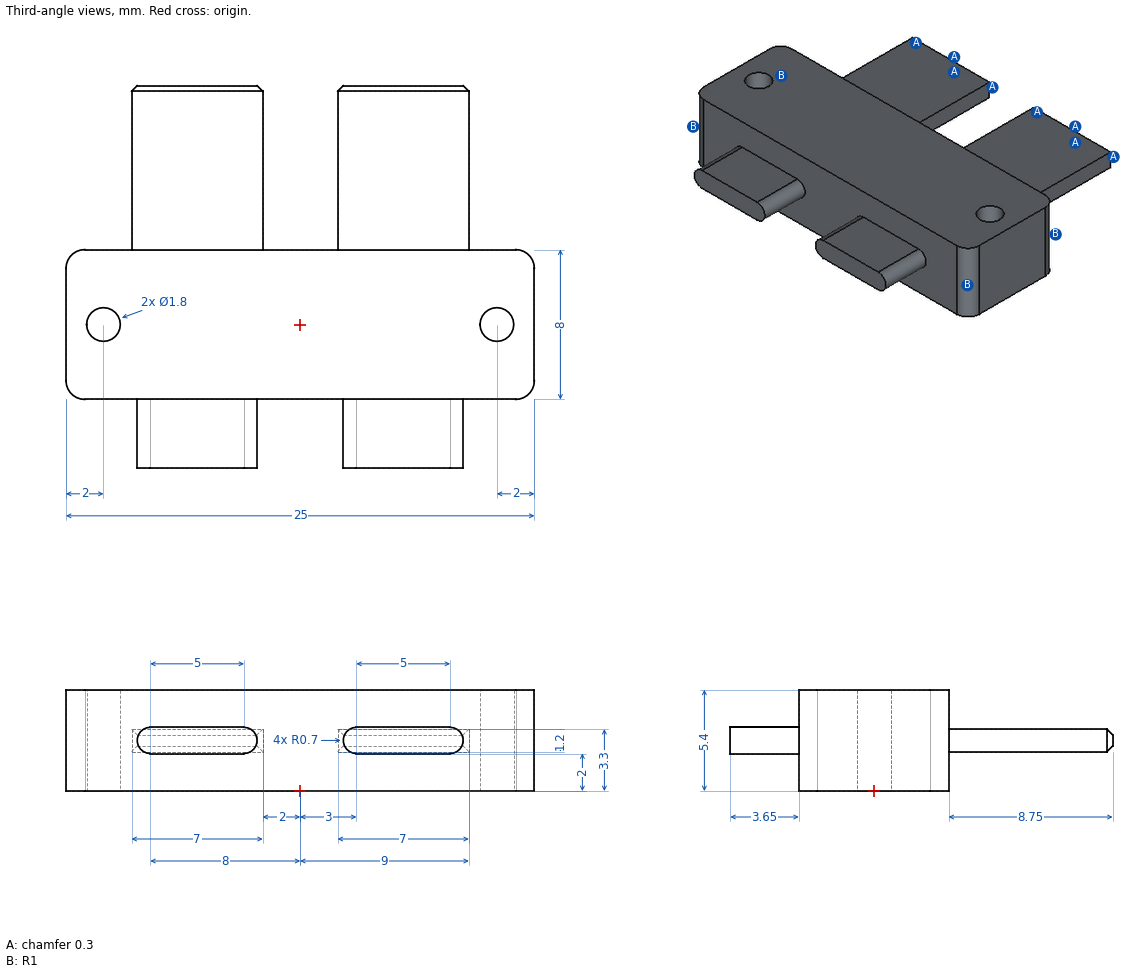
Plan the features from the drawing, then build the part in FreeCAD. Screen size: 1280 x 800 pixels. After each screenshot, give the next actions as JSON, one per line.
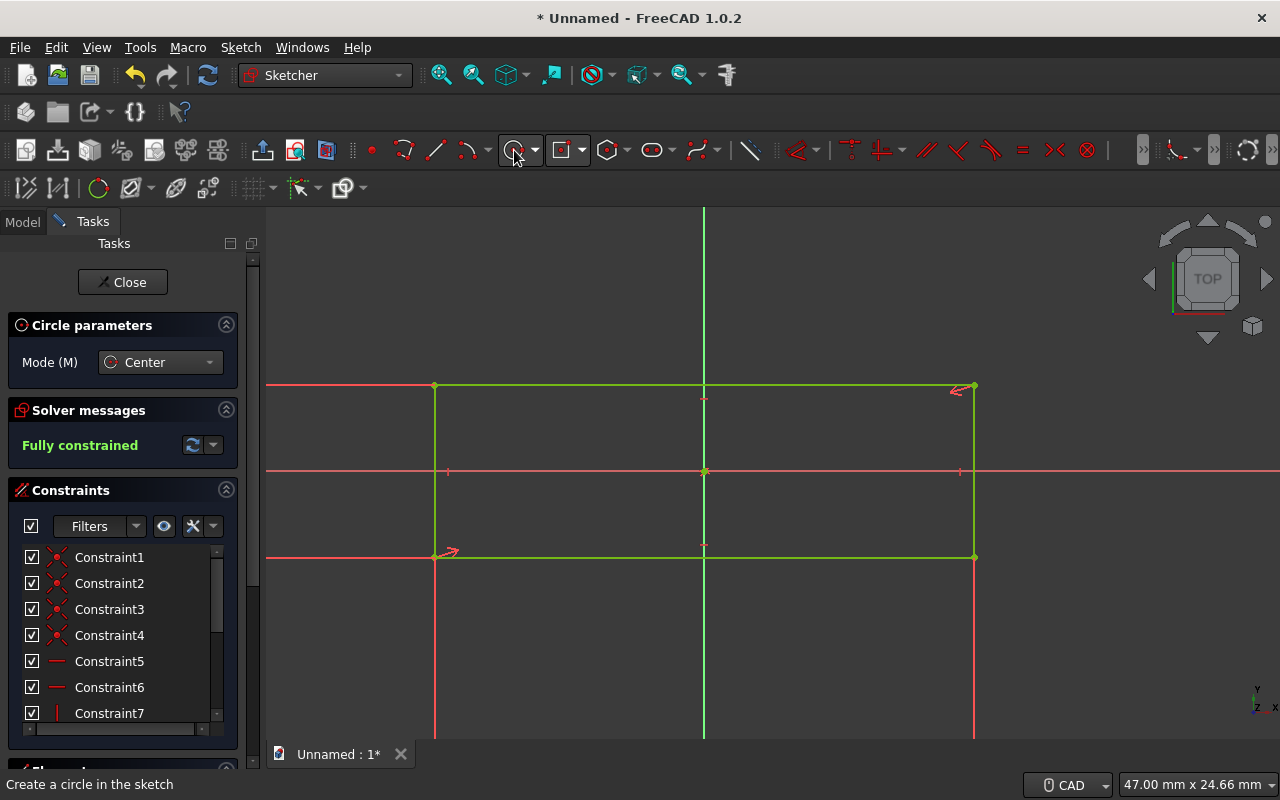
{"action": "left_click", "coordinate": [478, 471]}
{"action": "mouse_move", "coordinate": [485, 453]}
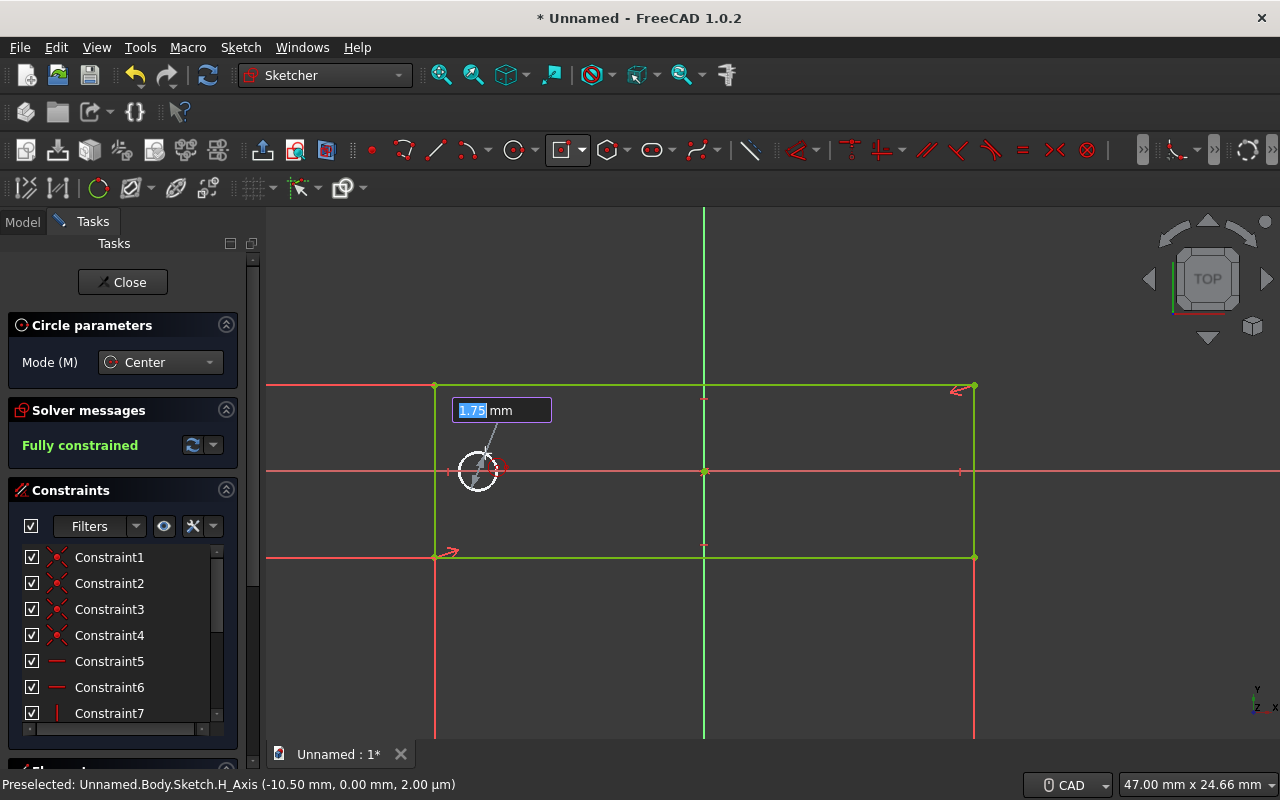
{"action": "type", "text": "1.8"}
{"action": "key", "text": "Return"}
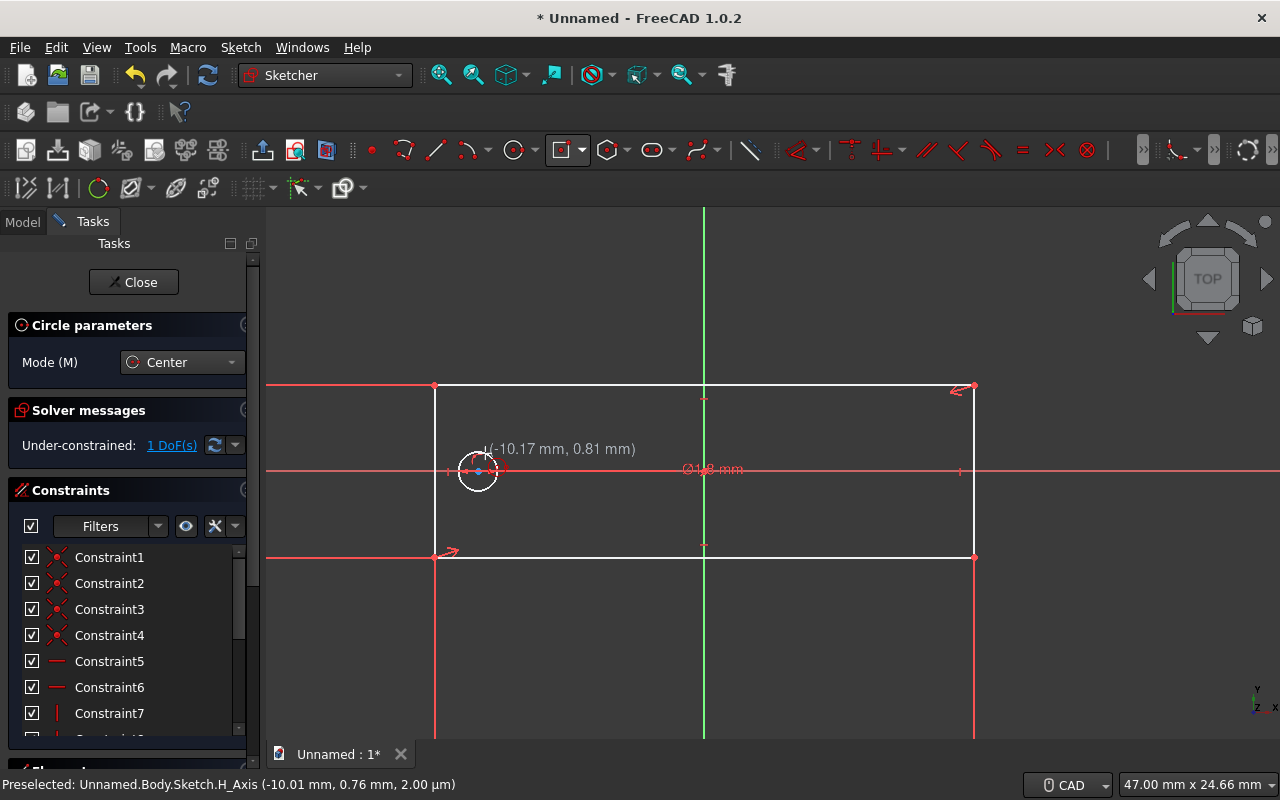
{"action": "left_click", "coordinate": [931, 471]}
{"action": "mouse_move", "coordinate": [938, 453]}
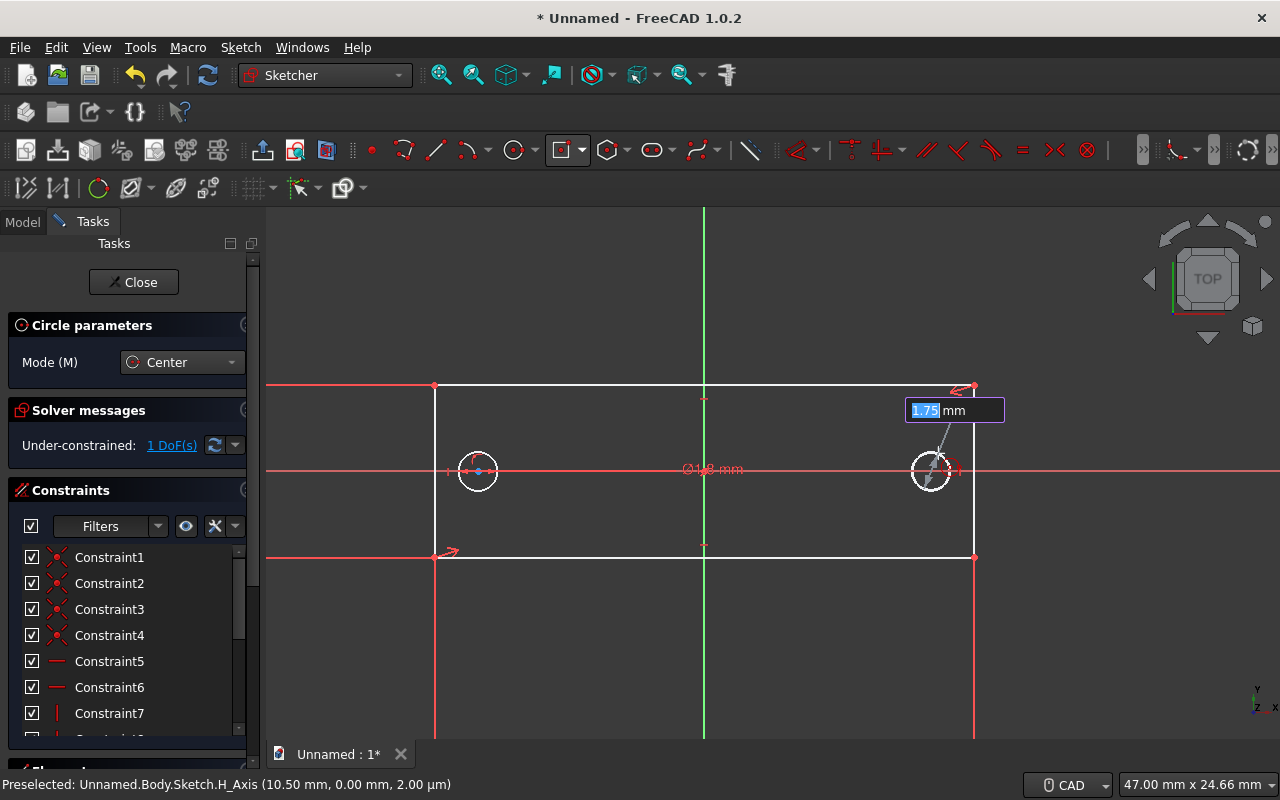
{"action": "type", "text": "1.8"}
{"action": "key", "text": "Return"}
{"action": "key", "text": "Escape"}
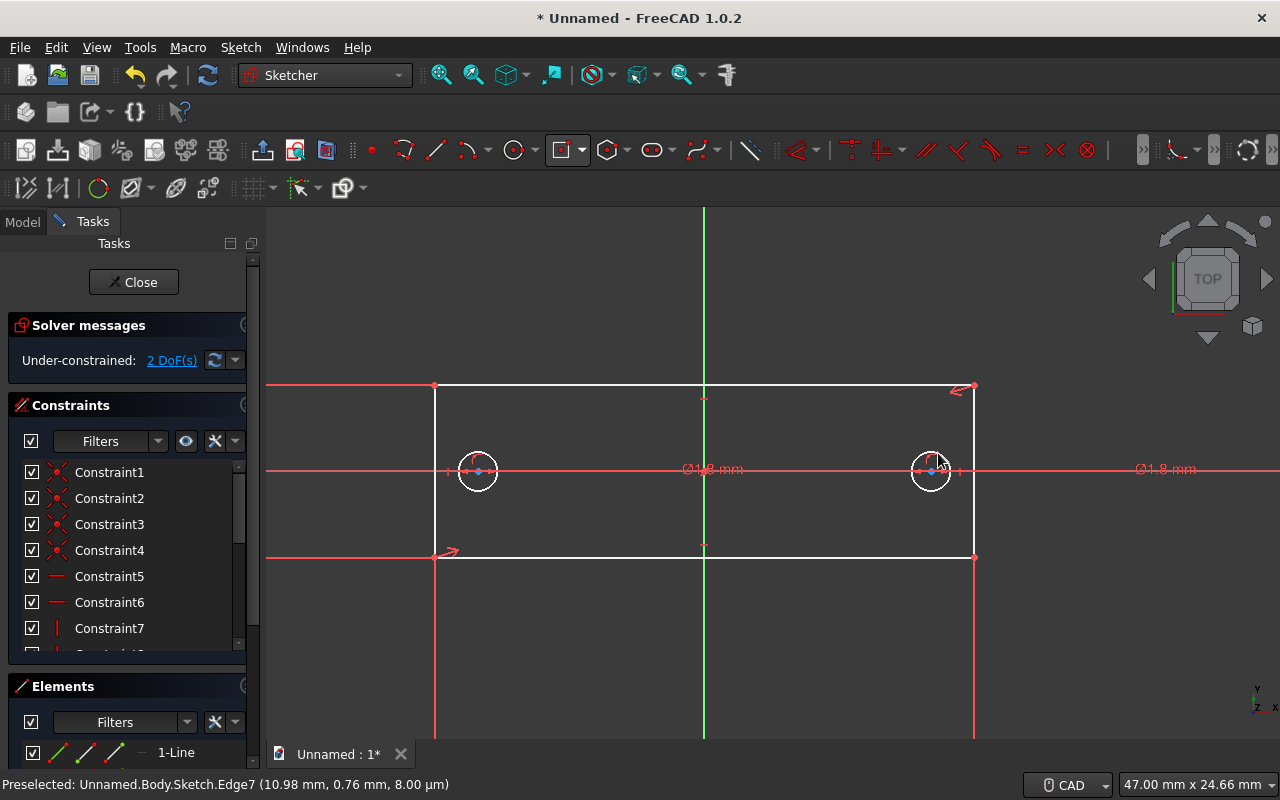
{"action": "left_click", "coordinate": [435, 558]}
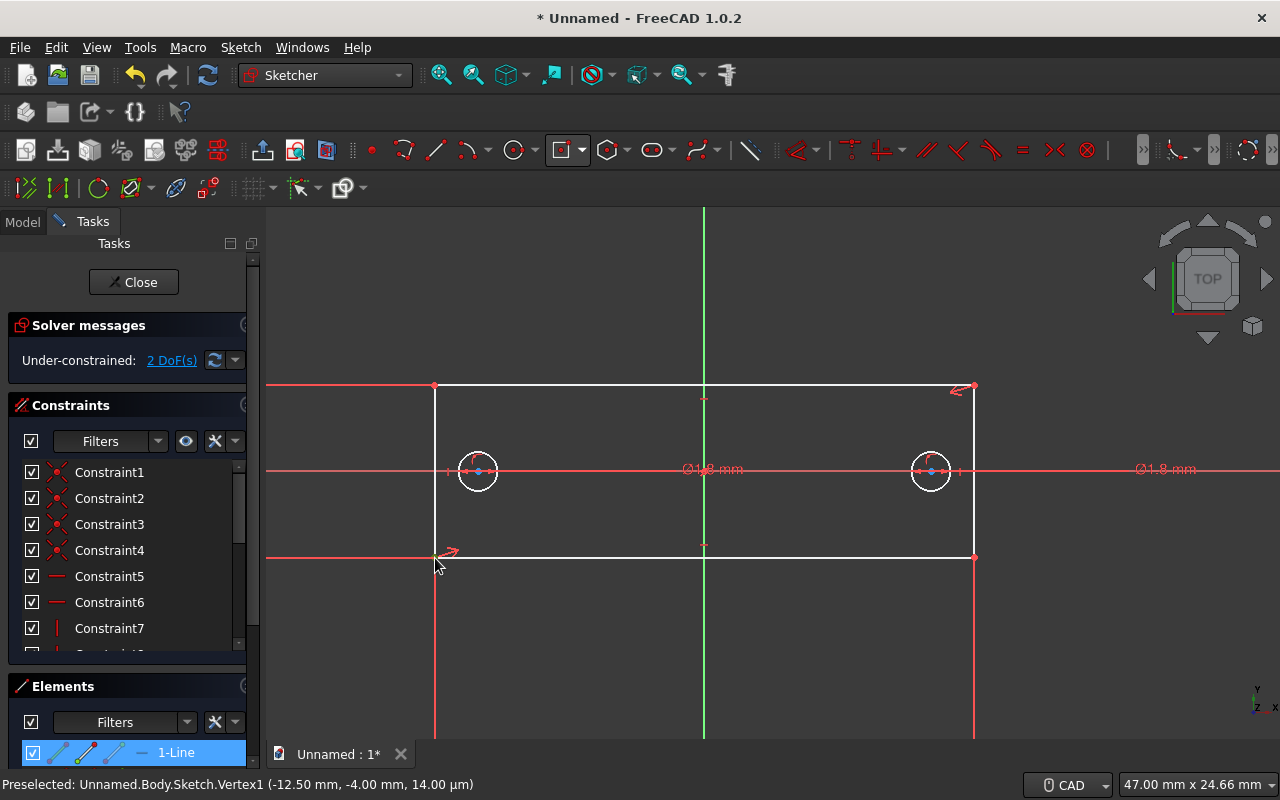
{"action": "left_click", "coordinate": [478, 471]}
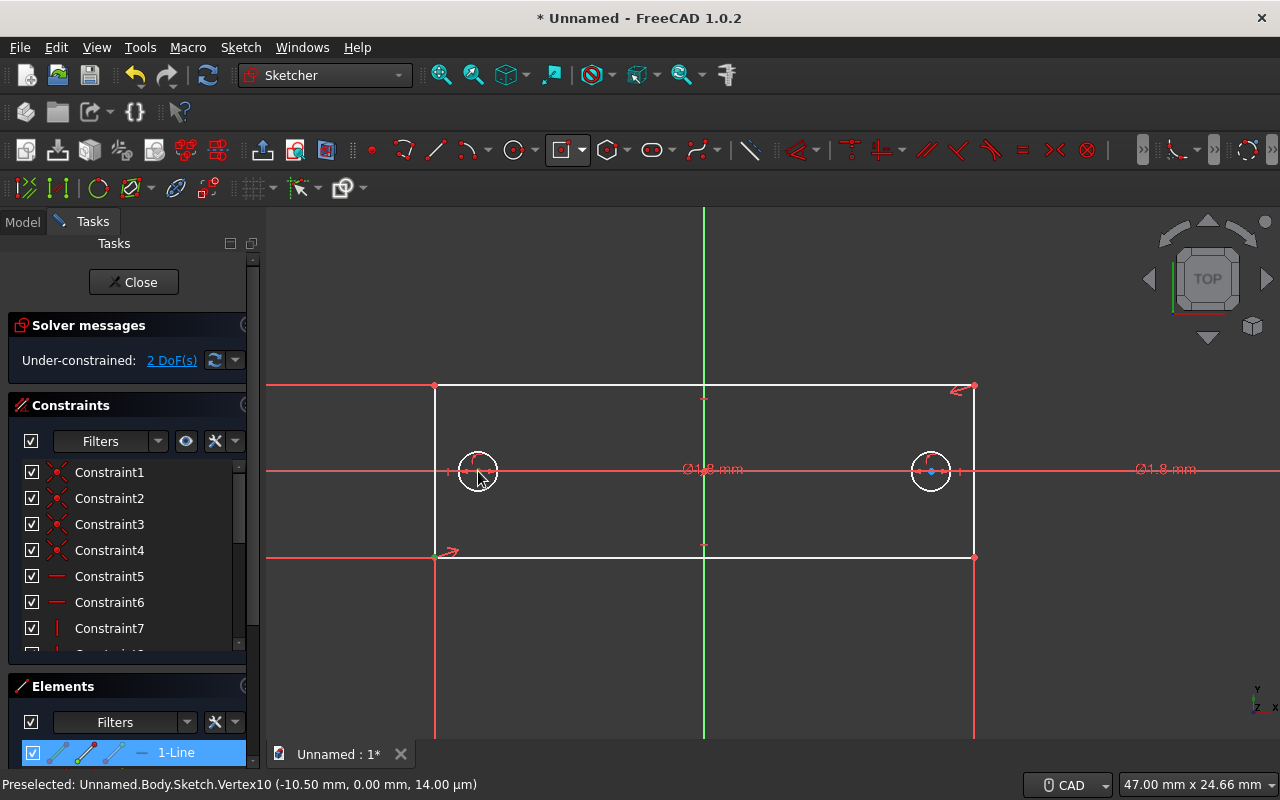
{"action": "left_click", "coordinate": [818, 150]}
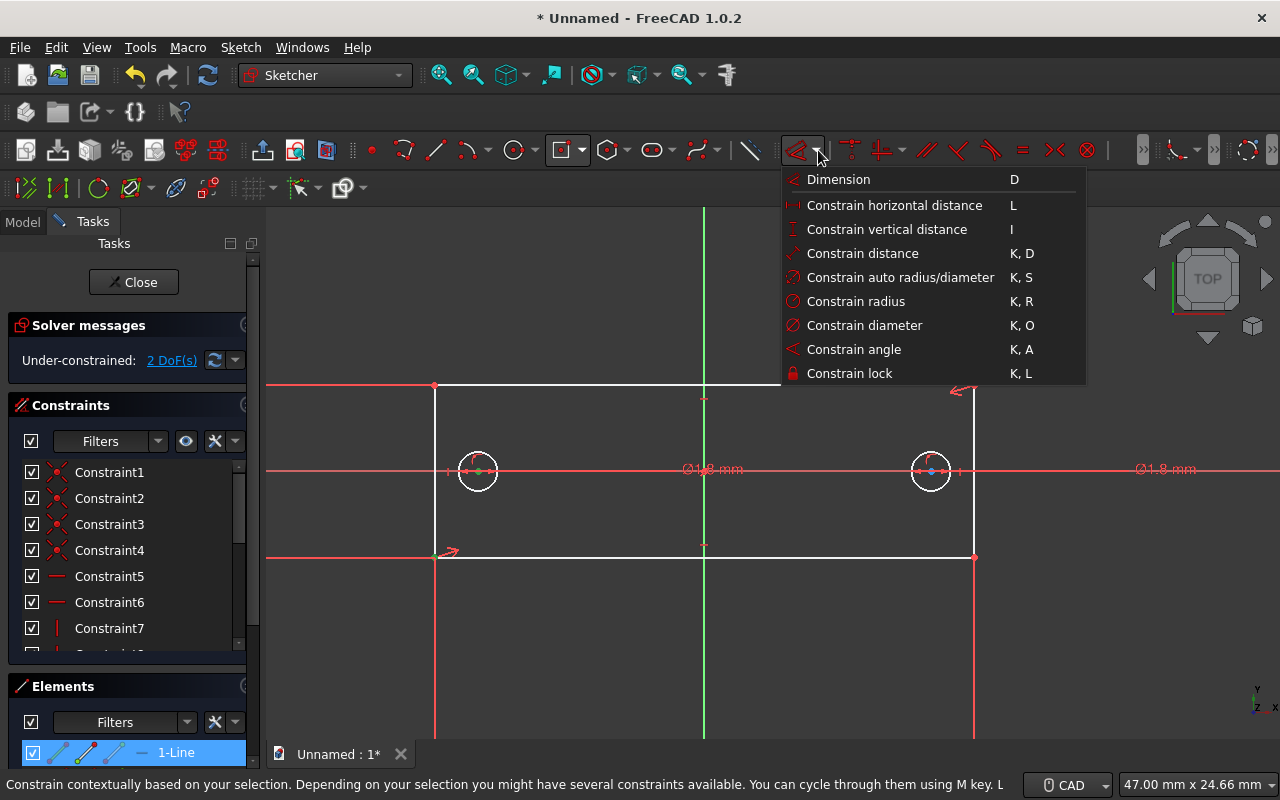
{"action": "left_click", "coordinate": [934, 205]}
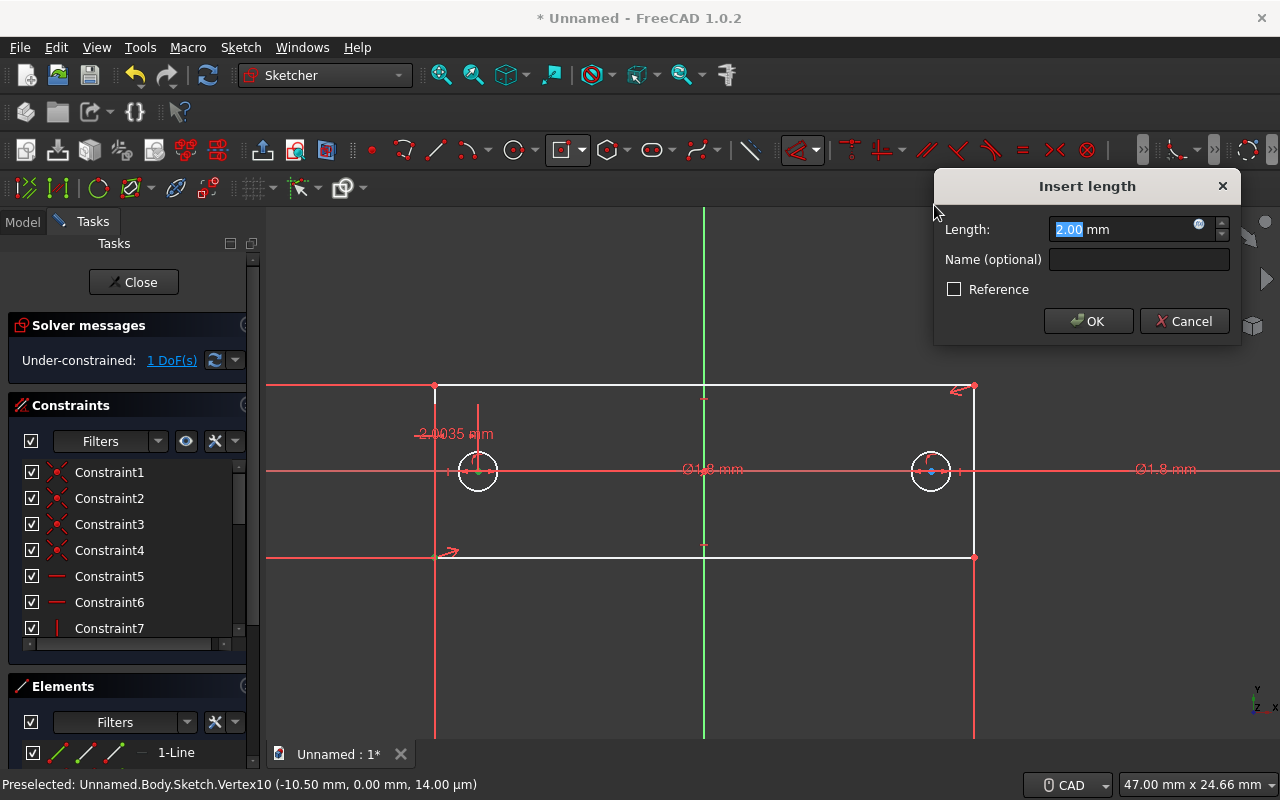
{"action": "type", "text": "2"}
{"action": "key", "text": "Return"}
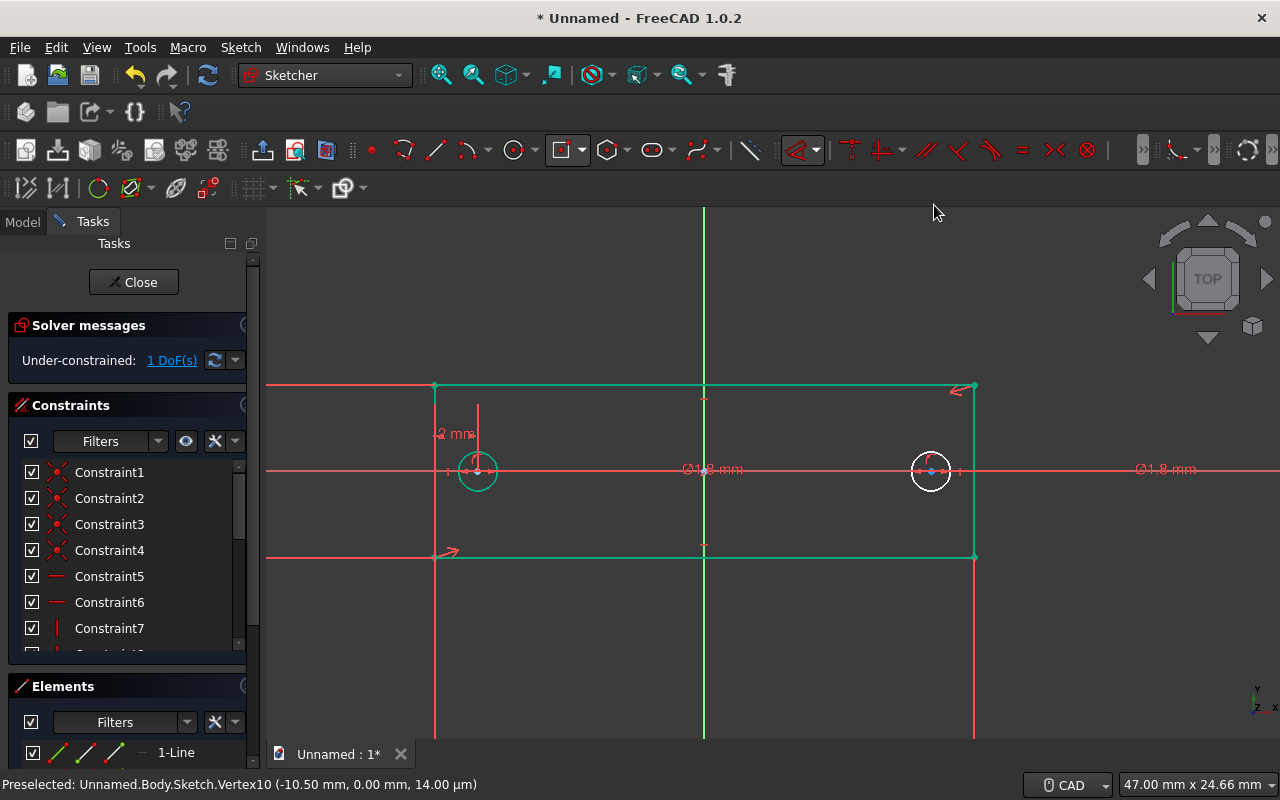
{"action": "left_click", "coordinate": [974, 558]}